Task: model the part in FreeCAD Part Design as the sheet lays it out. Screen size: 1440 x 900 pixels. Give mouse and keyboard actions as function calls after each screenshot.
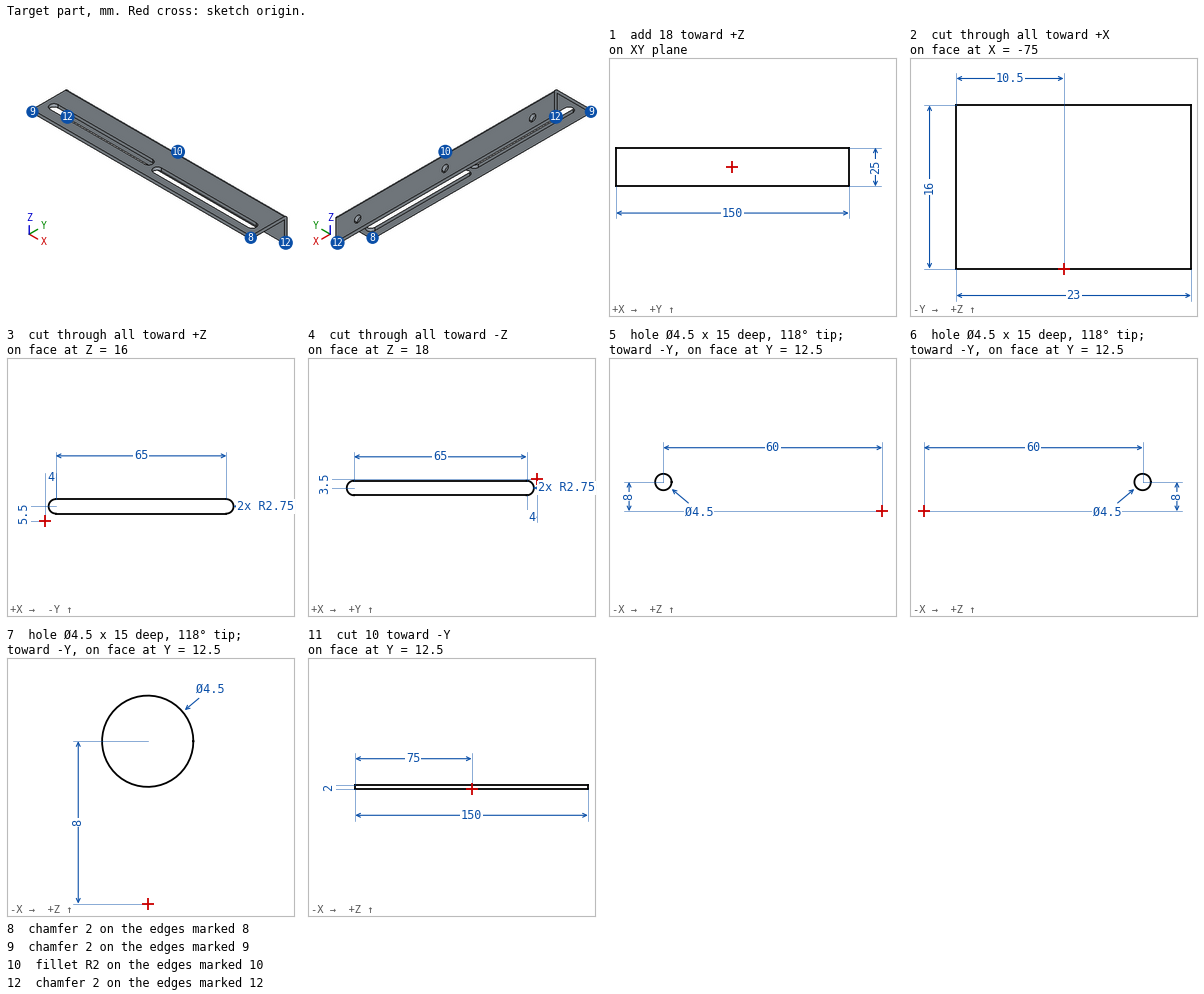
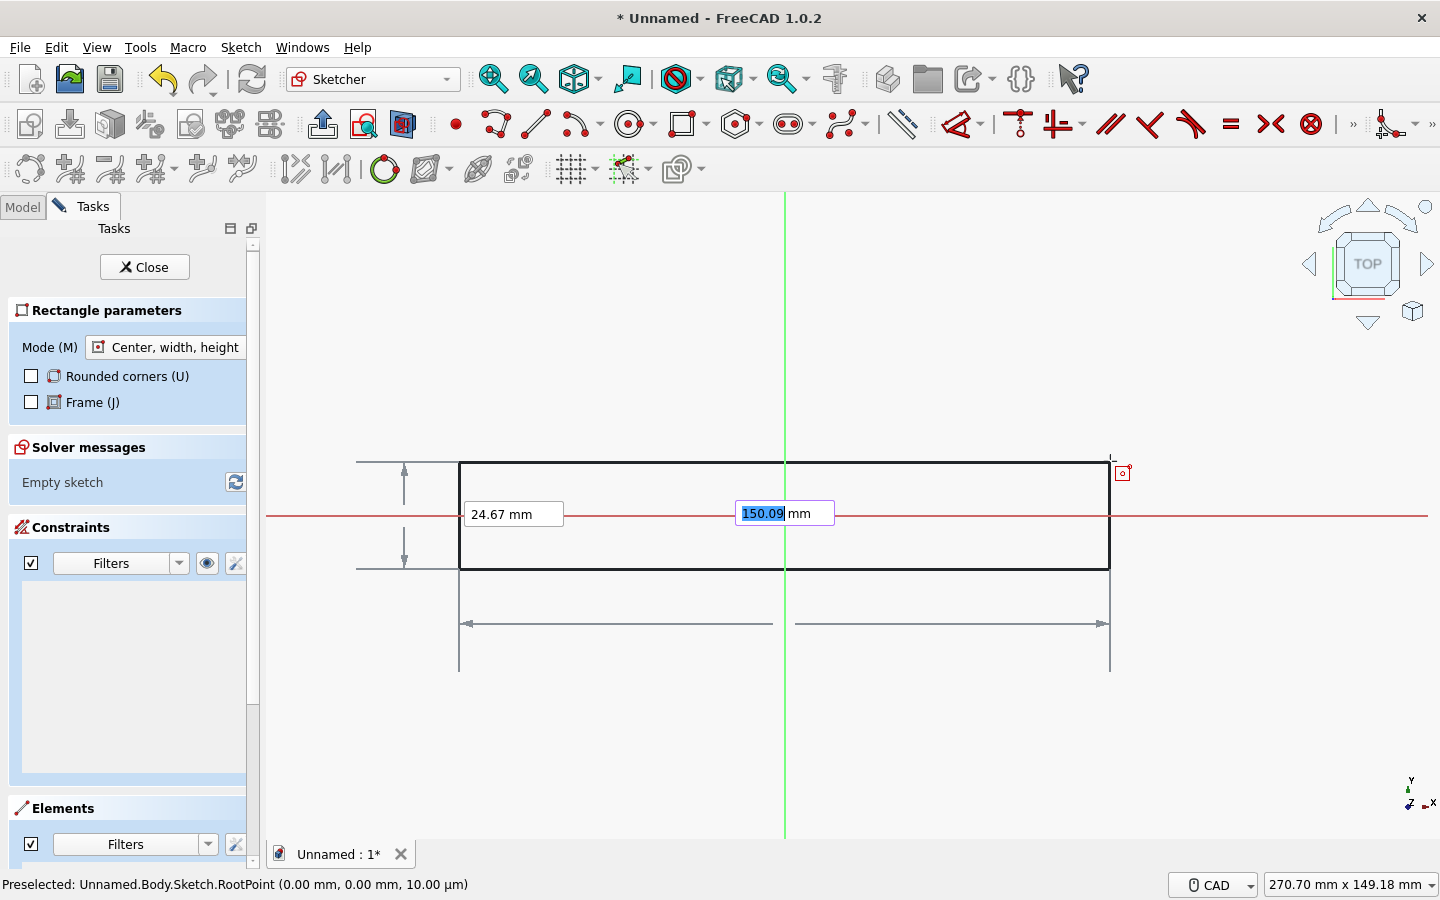
text(150)
key(Tab)
text(25)
key(Return)
key(Escape)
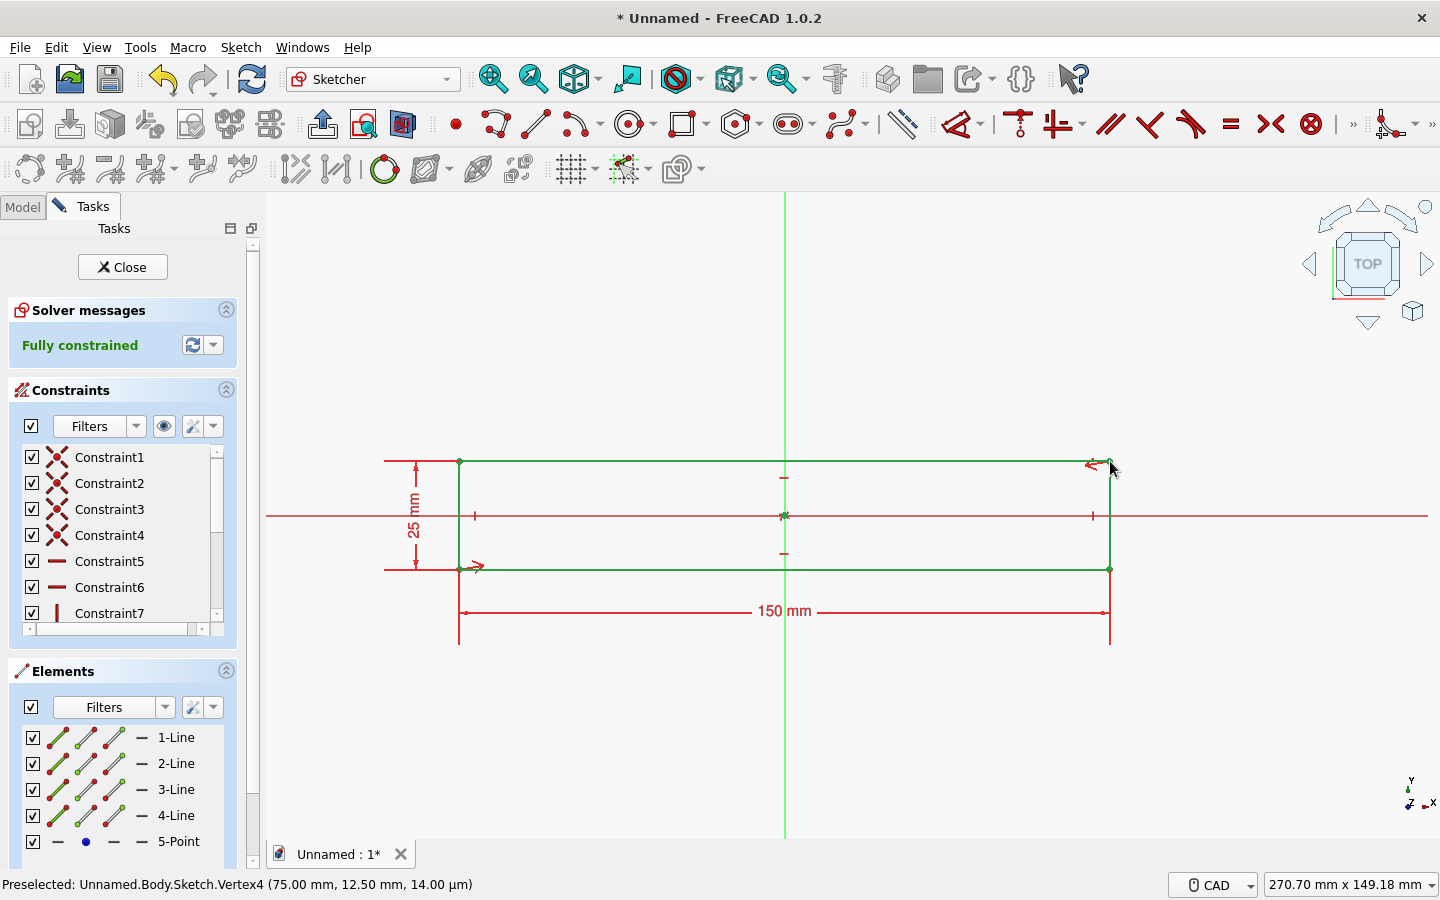
click(123, 267)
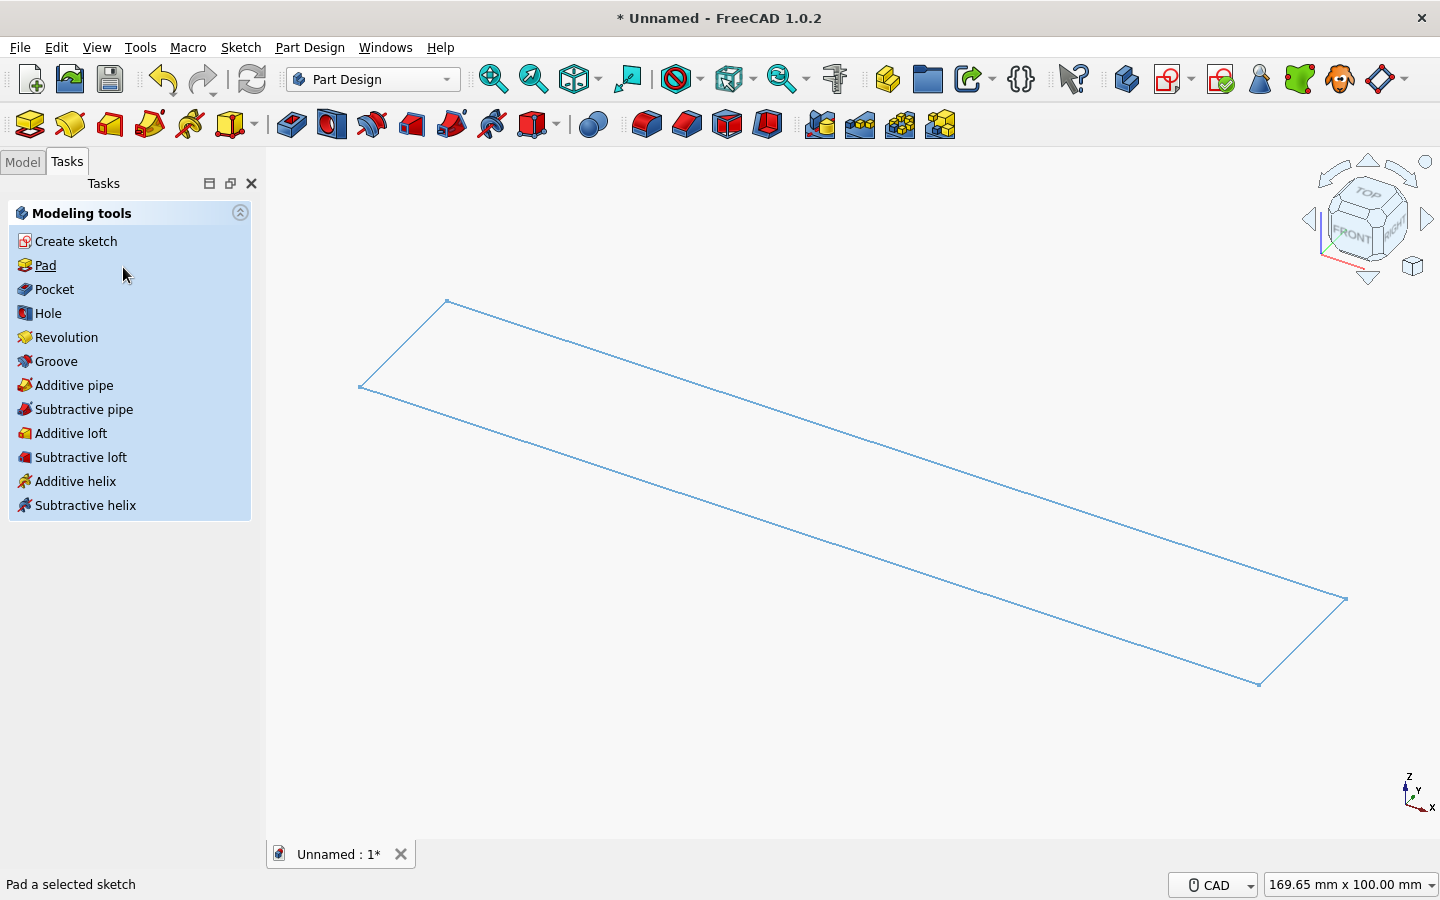
click(30, 124)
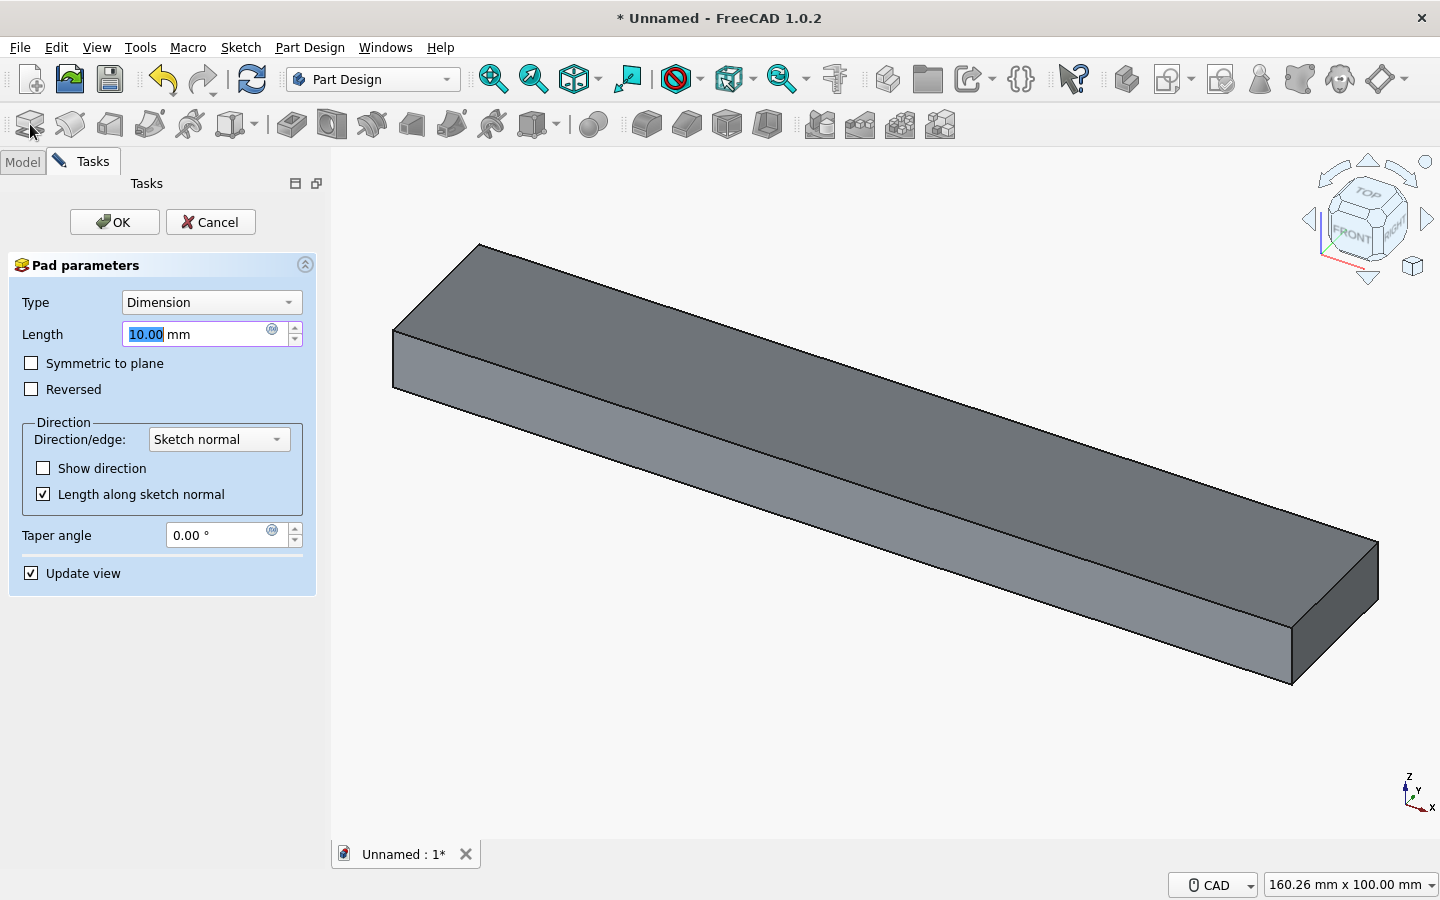
text(18)
key(Tab)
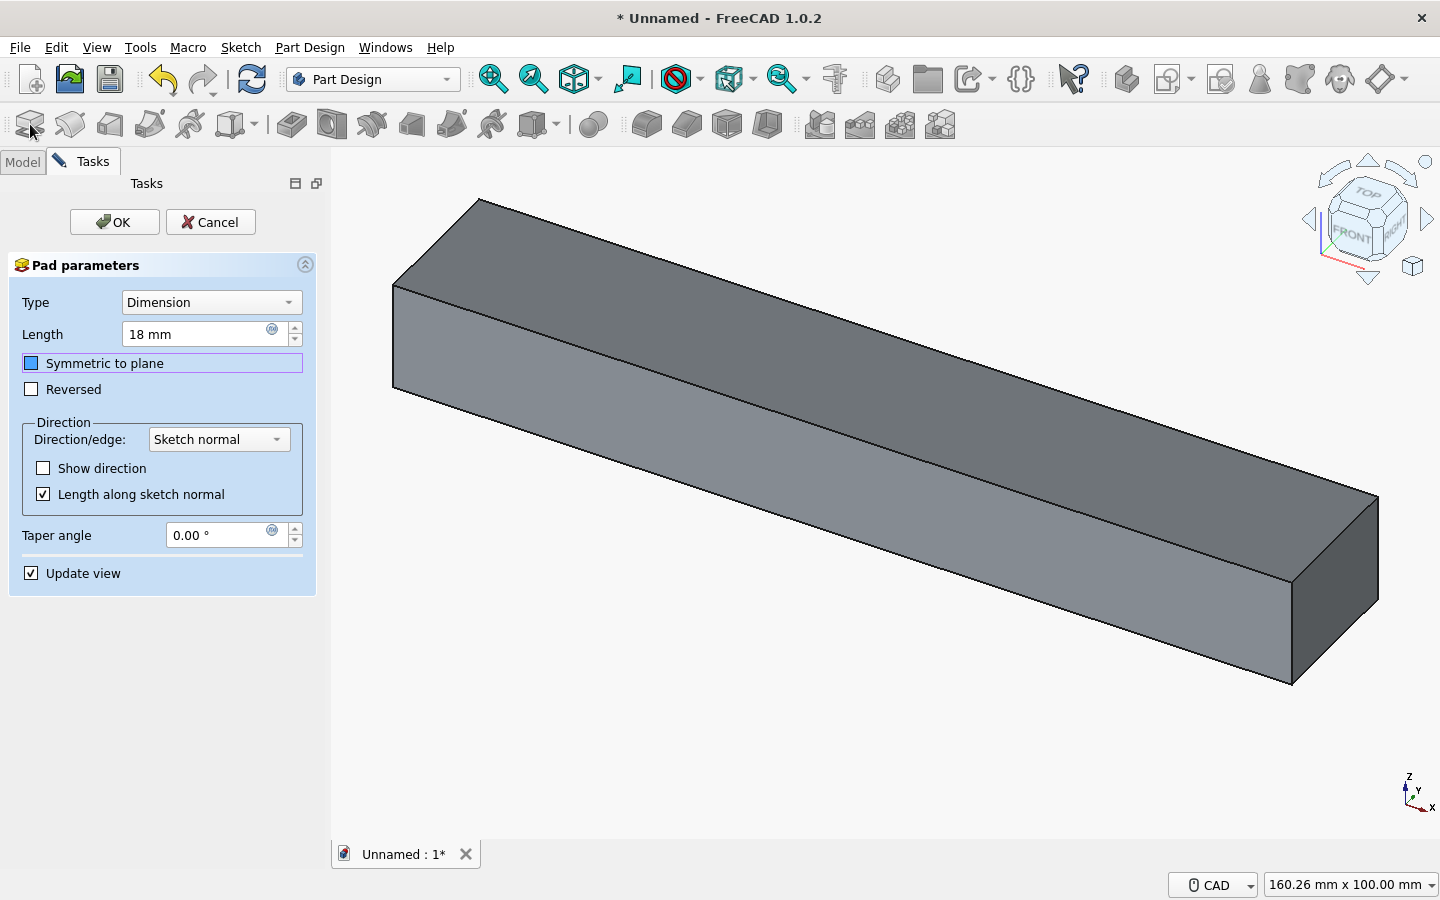
click(115, 222)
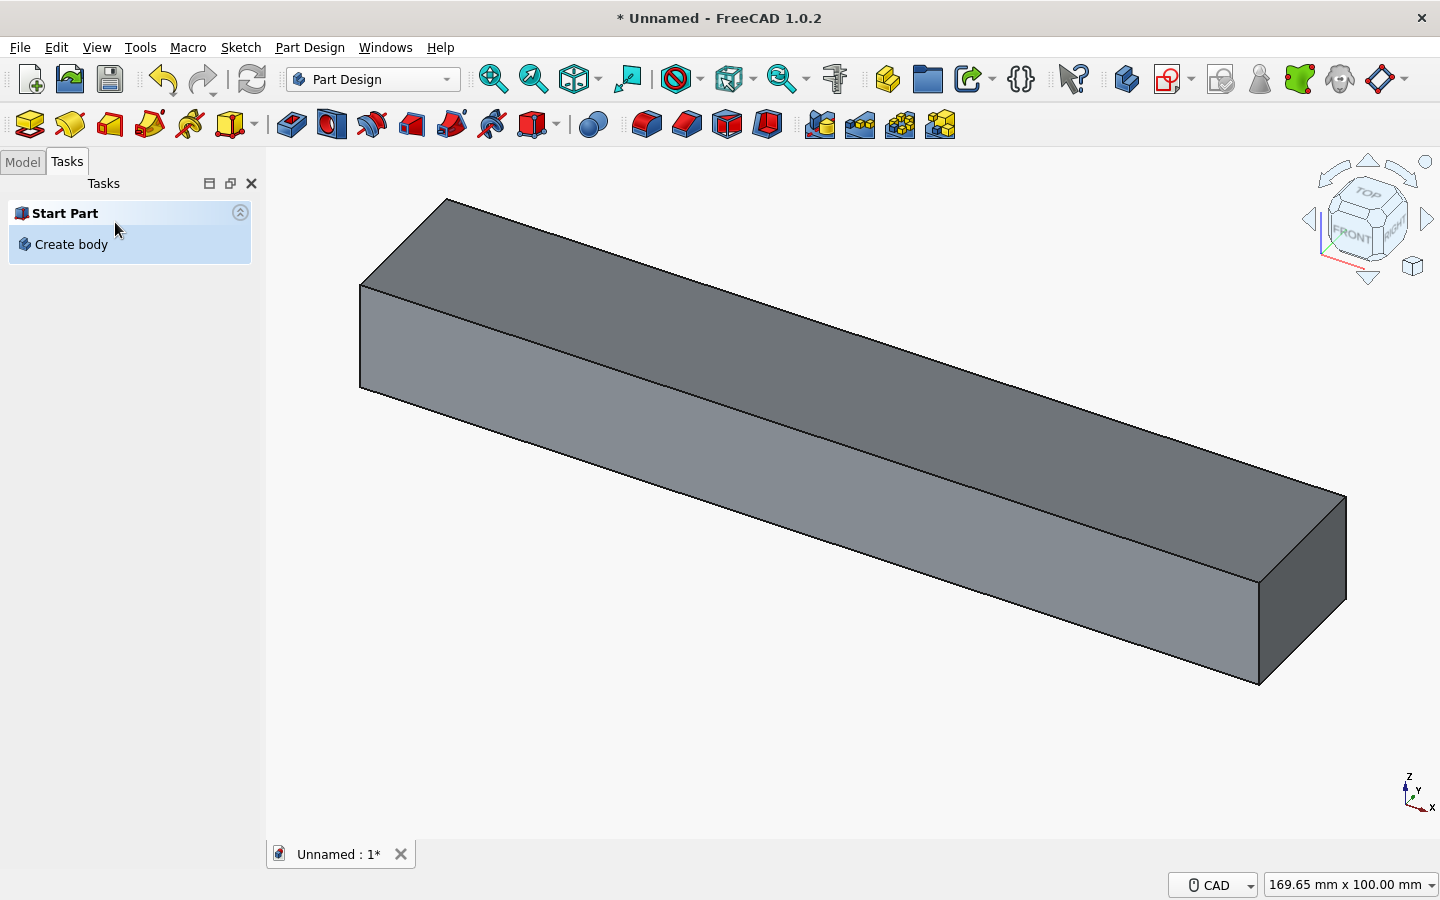
key(6)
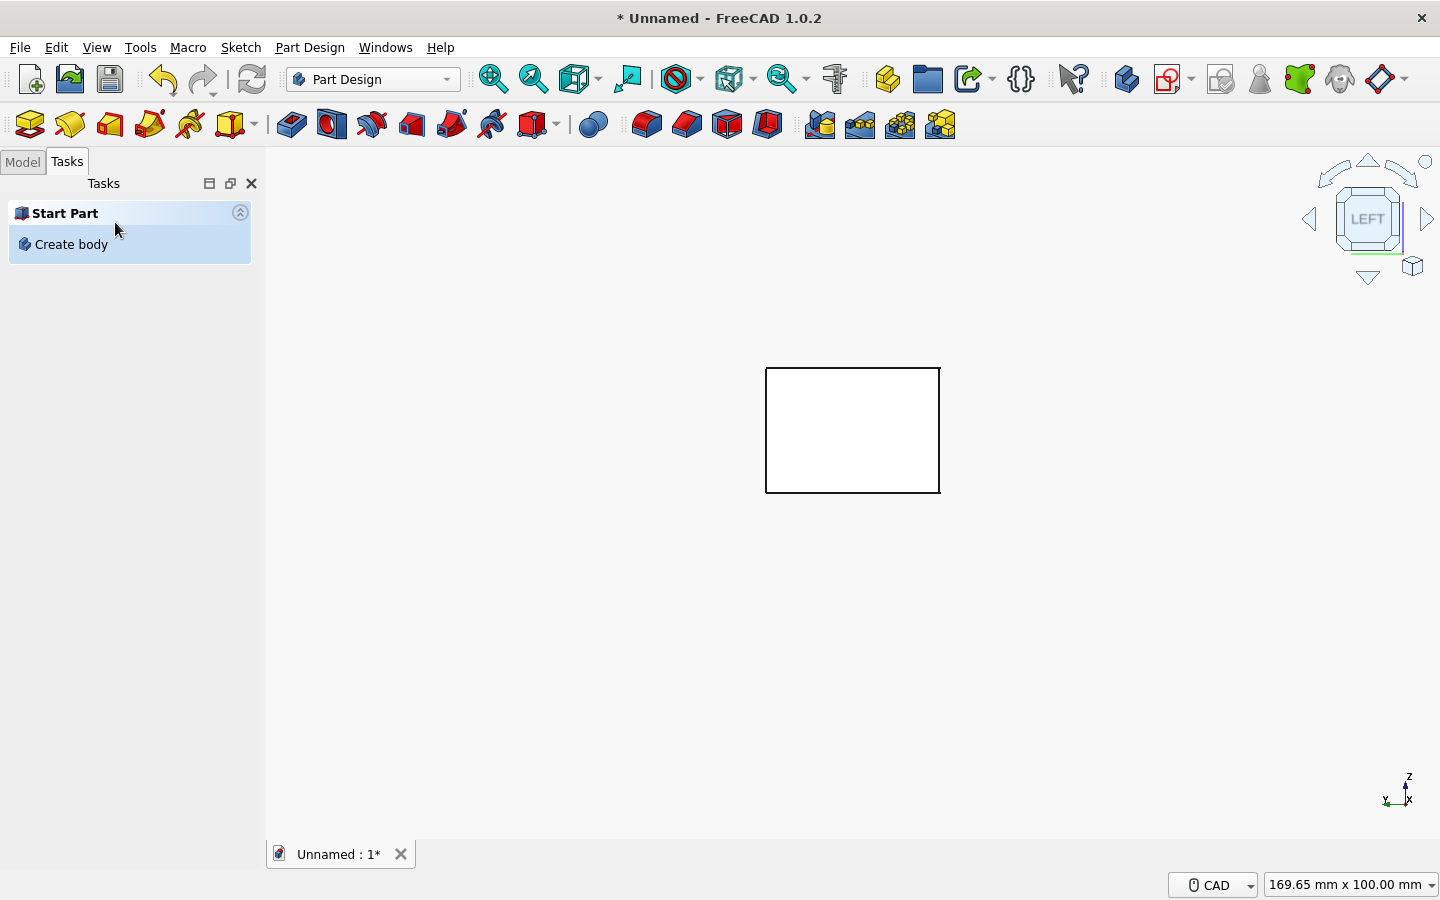
click(494, 80)